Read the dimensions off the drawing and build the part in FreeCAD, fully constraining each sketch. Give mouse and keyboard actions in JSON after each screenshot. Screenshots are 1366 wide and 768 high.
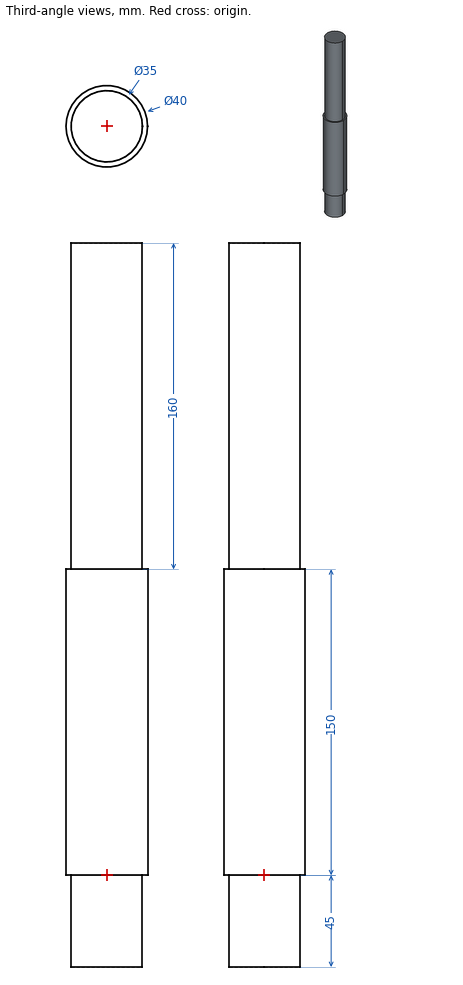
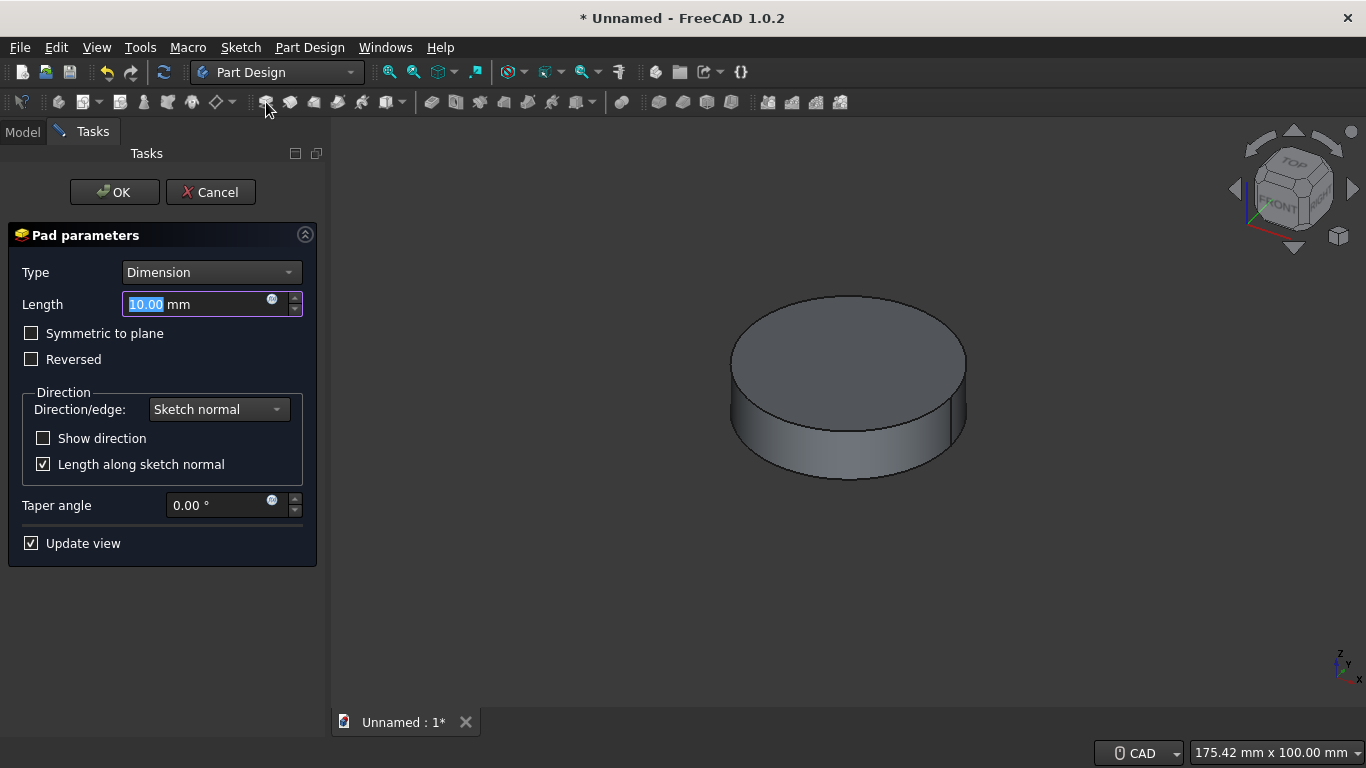
{"action": "type", "text": "150"}
{"action": "key", "text": "Tab"}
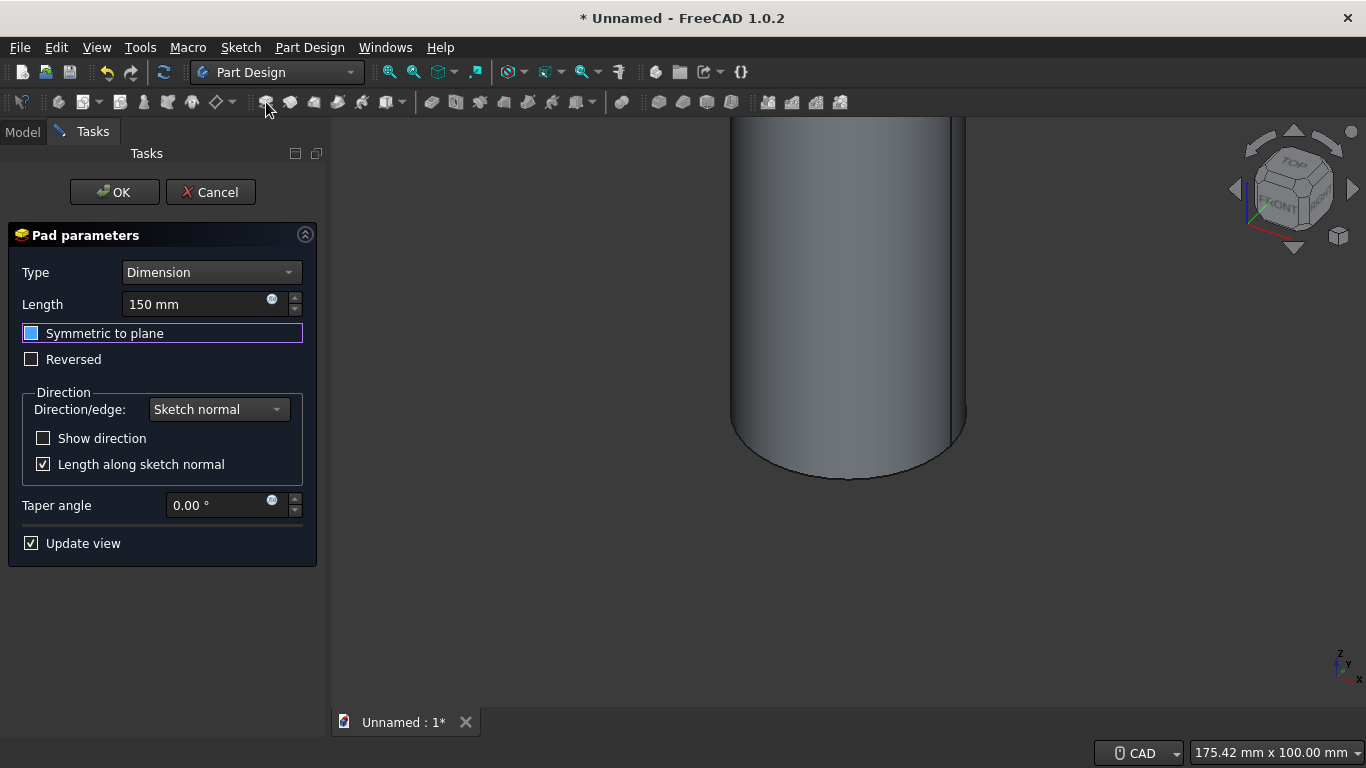
{"action": "left_click", "coordinate": [115, 192]}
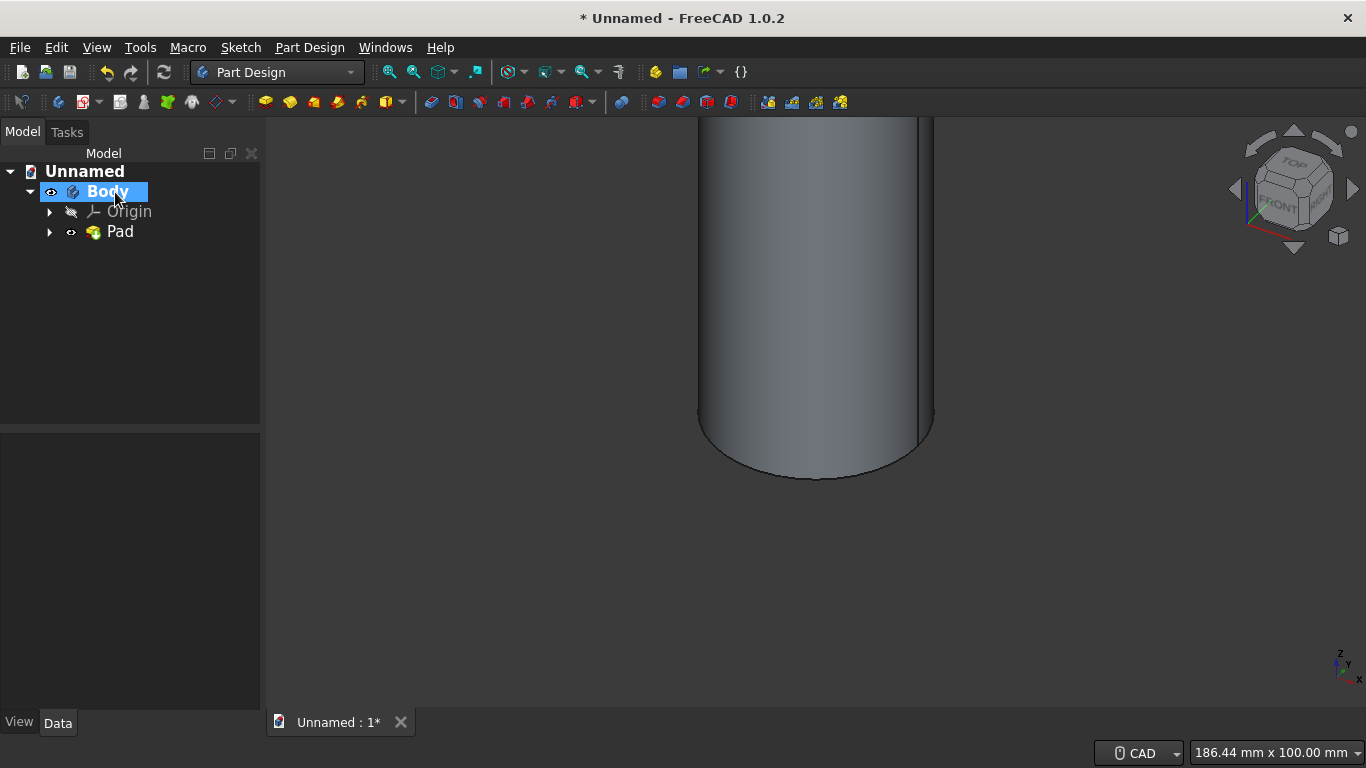
{"action": "key", "text": "v f"}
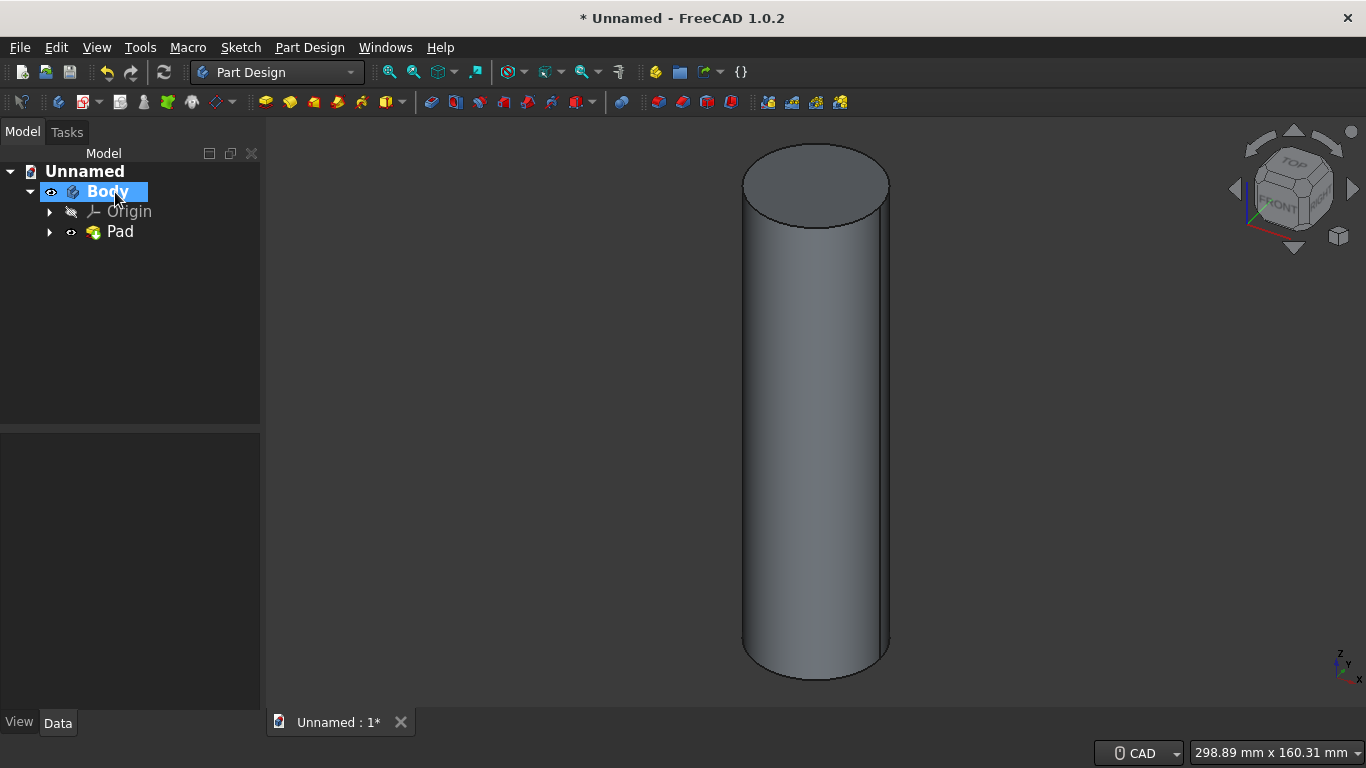
{"action": "left_click", "coordinate": [816, 185]}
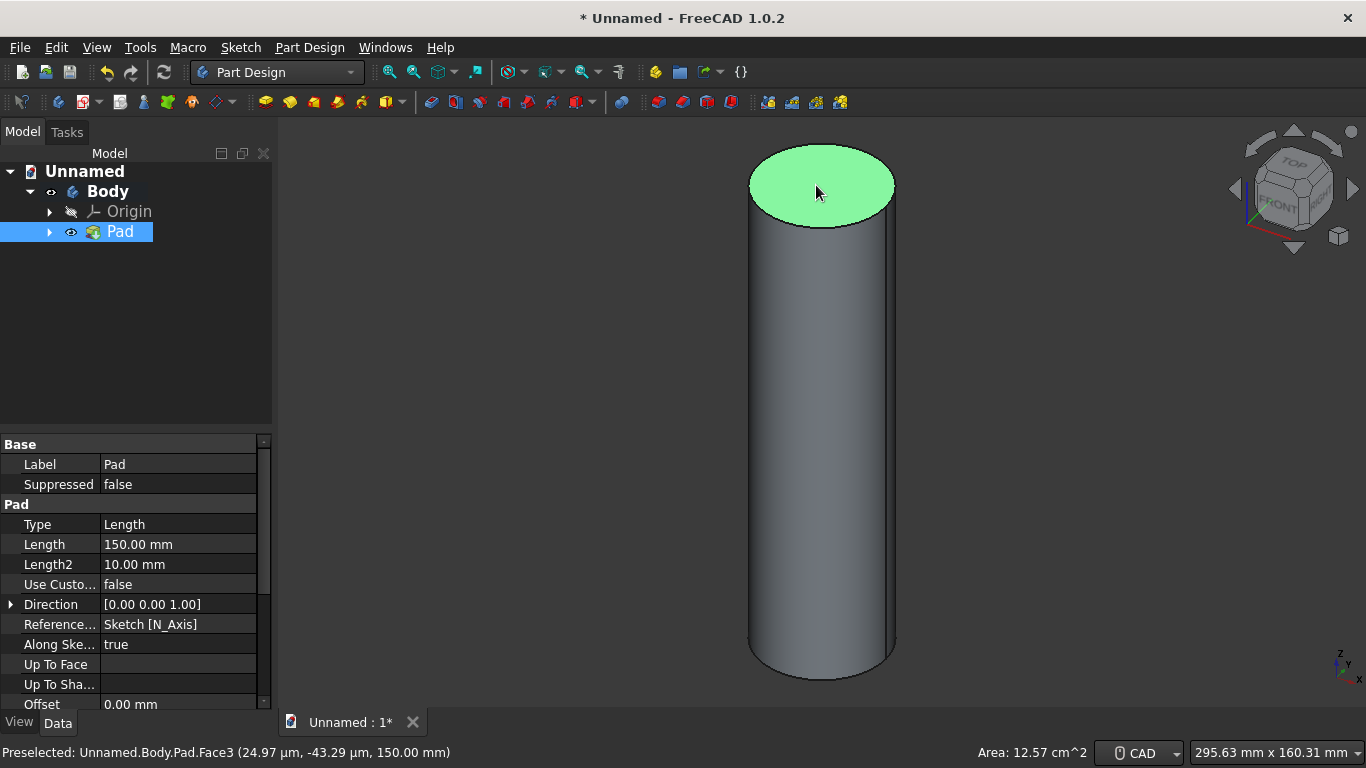
{"action": "left_click", "coordinate": [84, 102]}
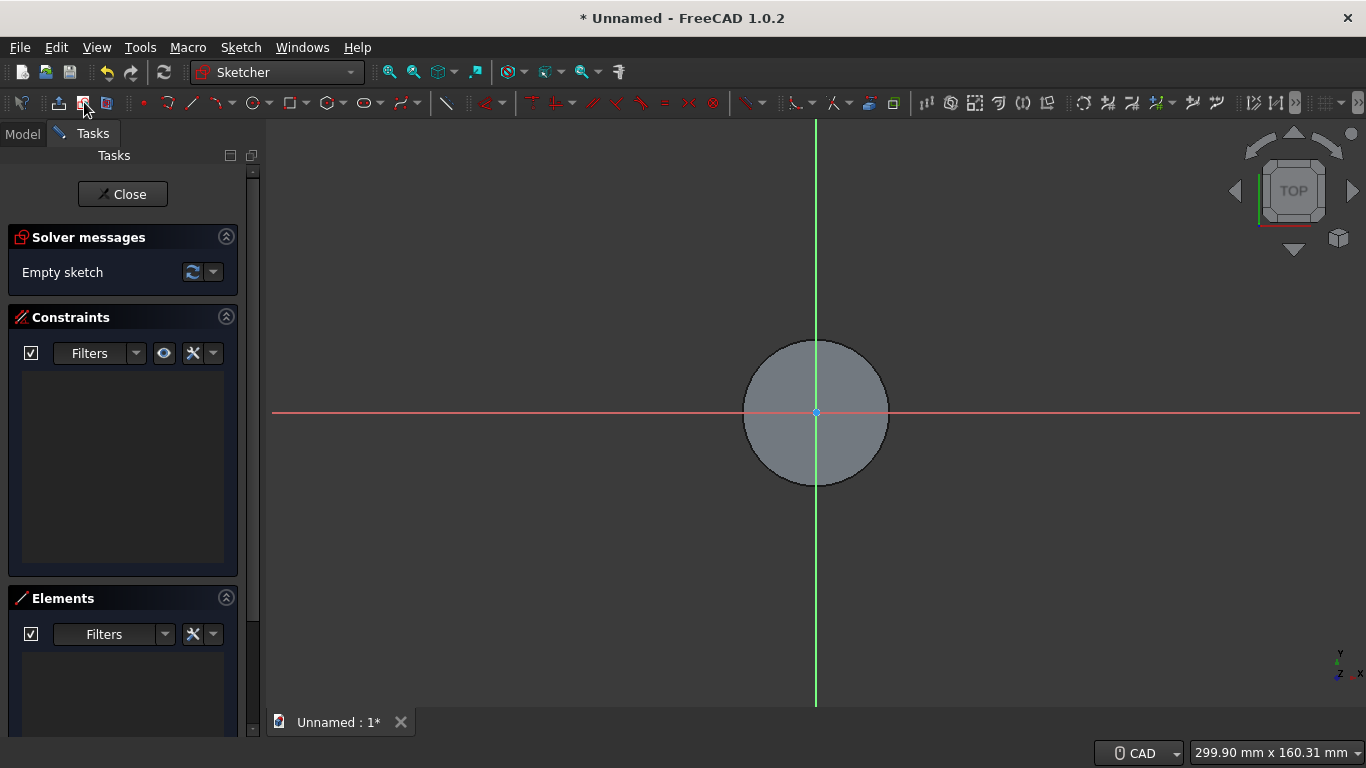
{"action": "scroll", "coordinate": [856, 413], "scroll_direction": "up", "scroll_amount": 5}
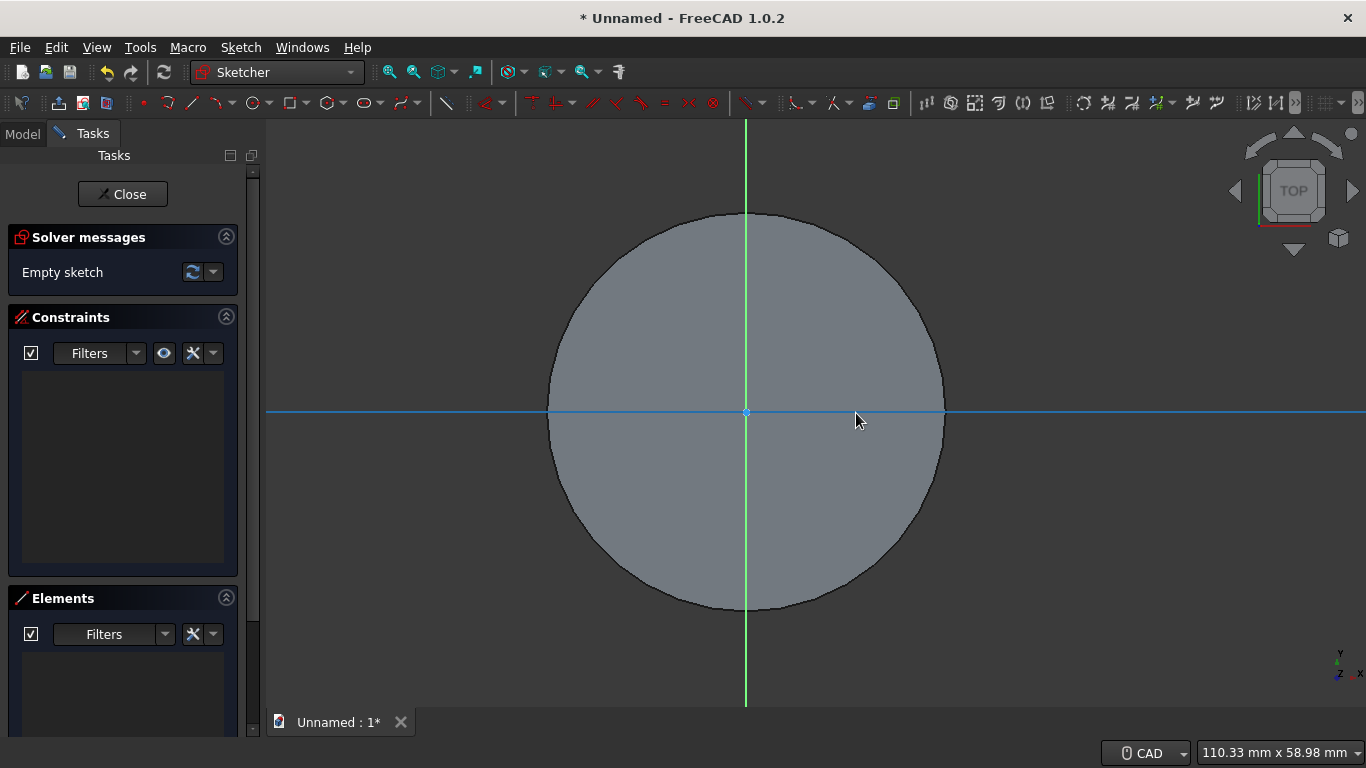
{"action": "key", "text": "g c"}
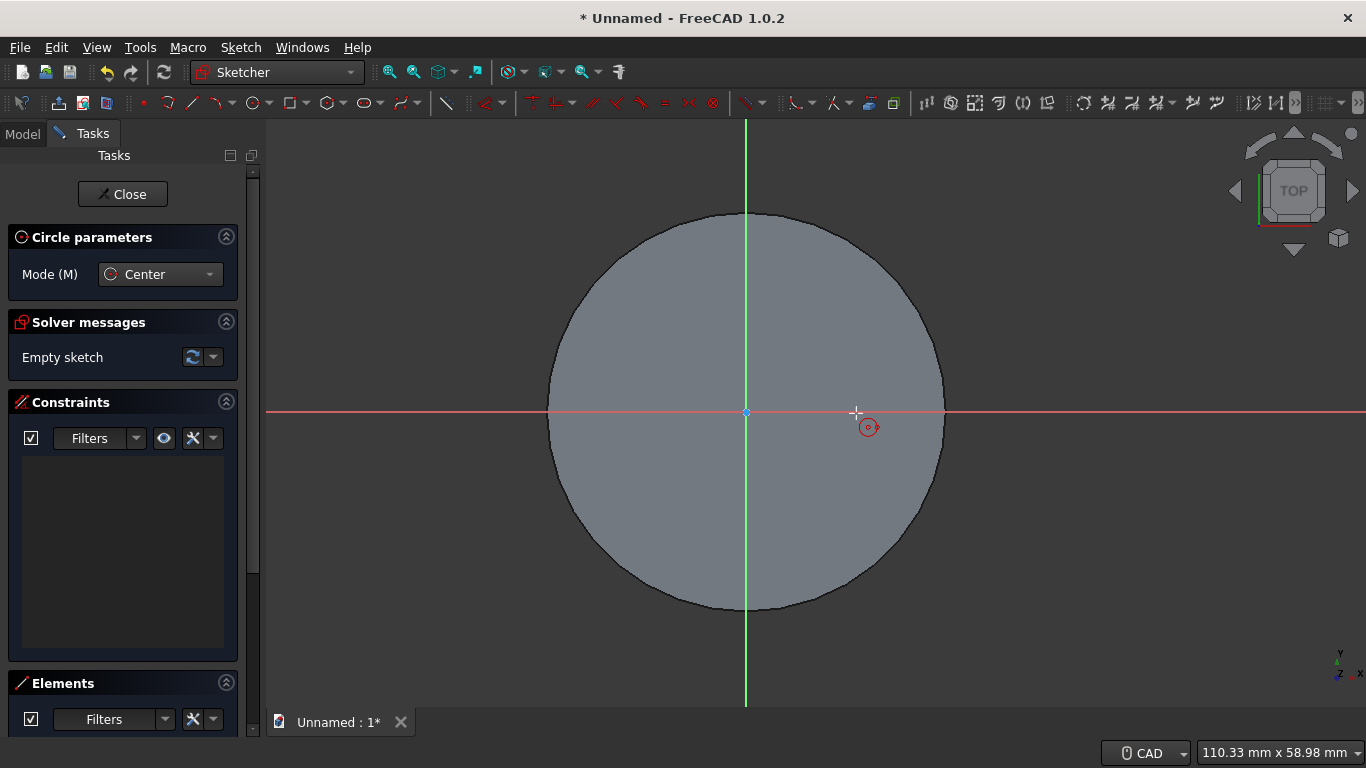
{"action": "left_click", "coordinate": [746, 412]}
{"action": "mouse_move", "coordinate": [870, 289]}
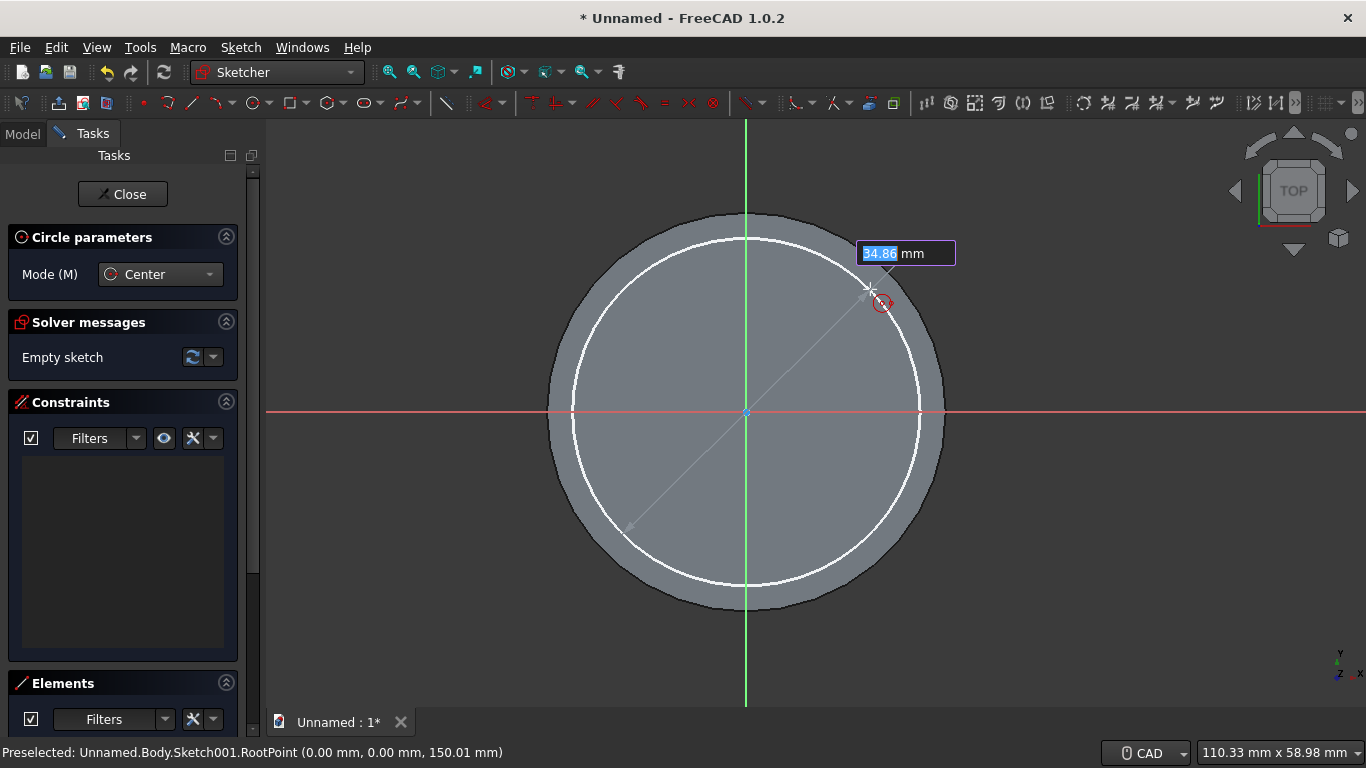
{"action": "type", "text": "35"}
{"action": "key", "text": "Return"}
{"action": "key", "text": "Escape"}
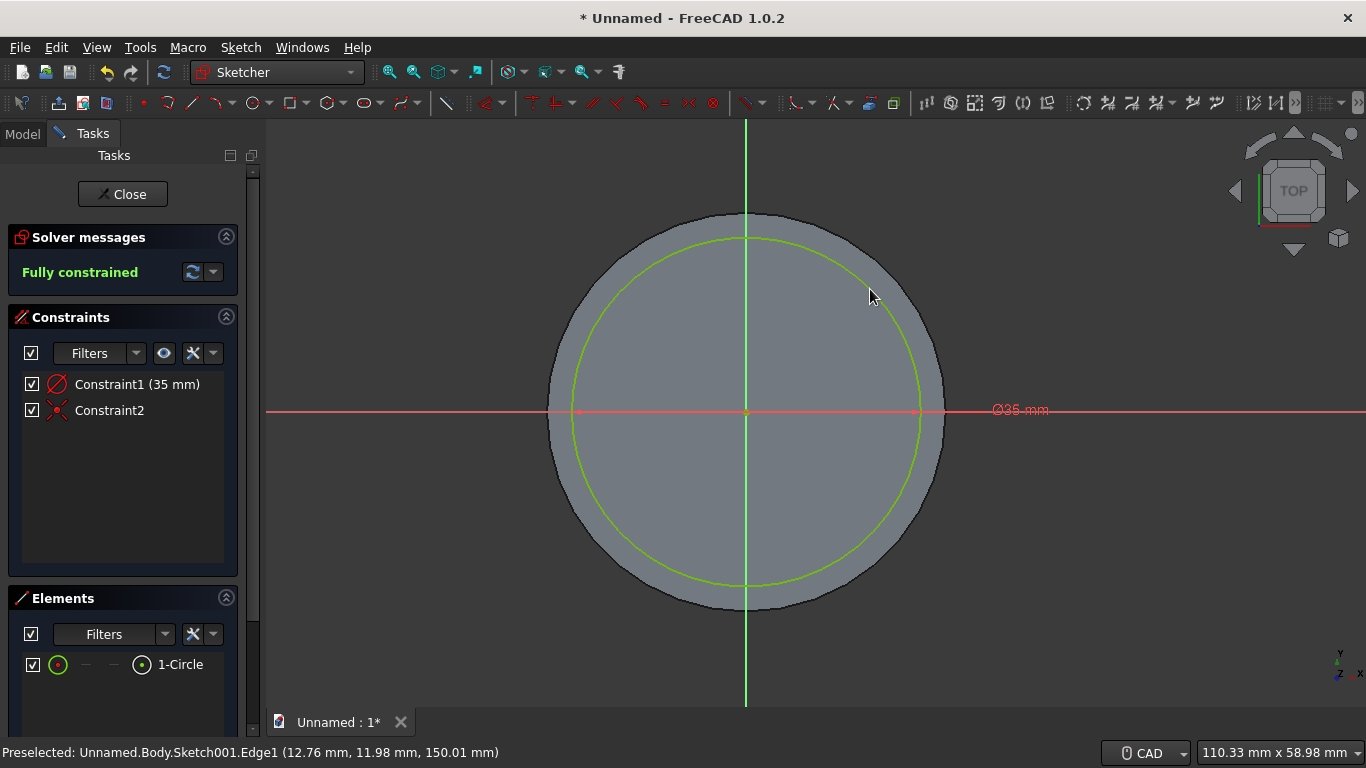
{"action": "left_click", "coordinate": [123, 194]}